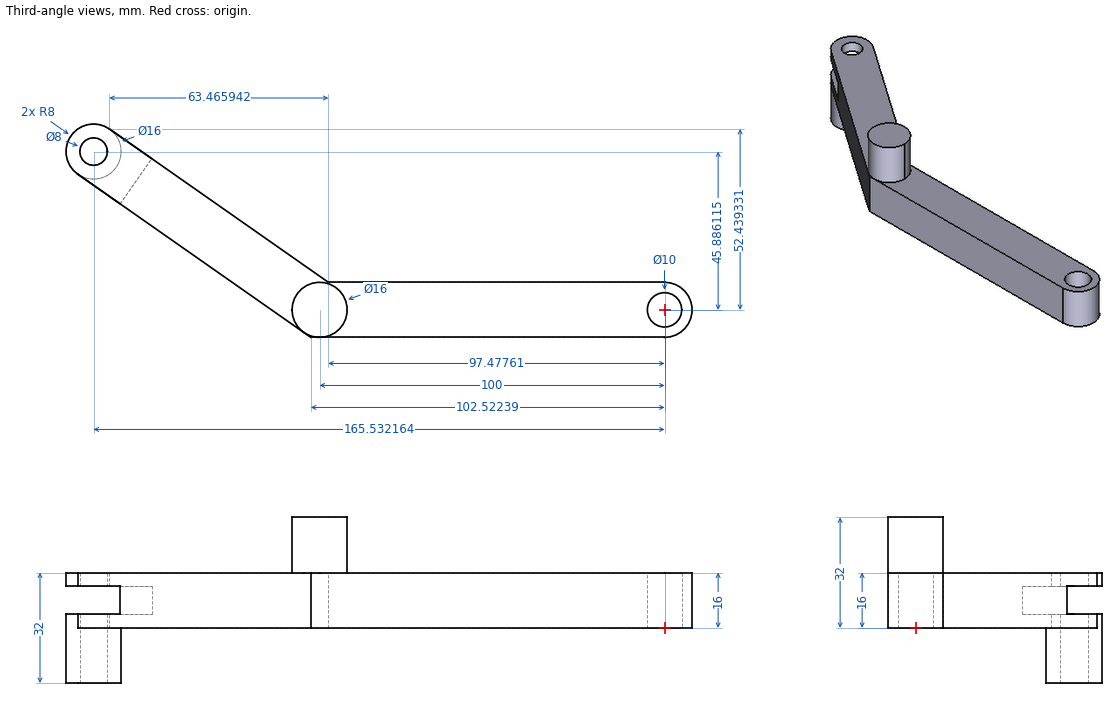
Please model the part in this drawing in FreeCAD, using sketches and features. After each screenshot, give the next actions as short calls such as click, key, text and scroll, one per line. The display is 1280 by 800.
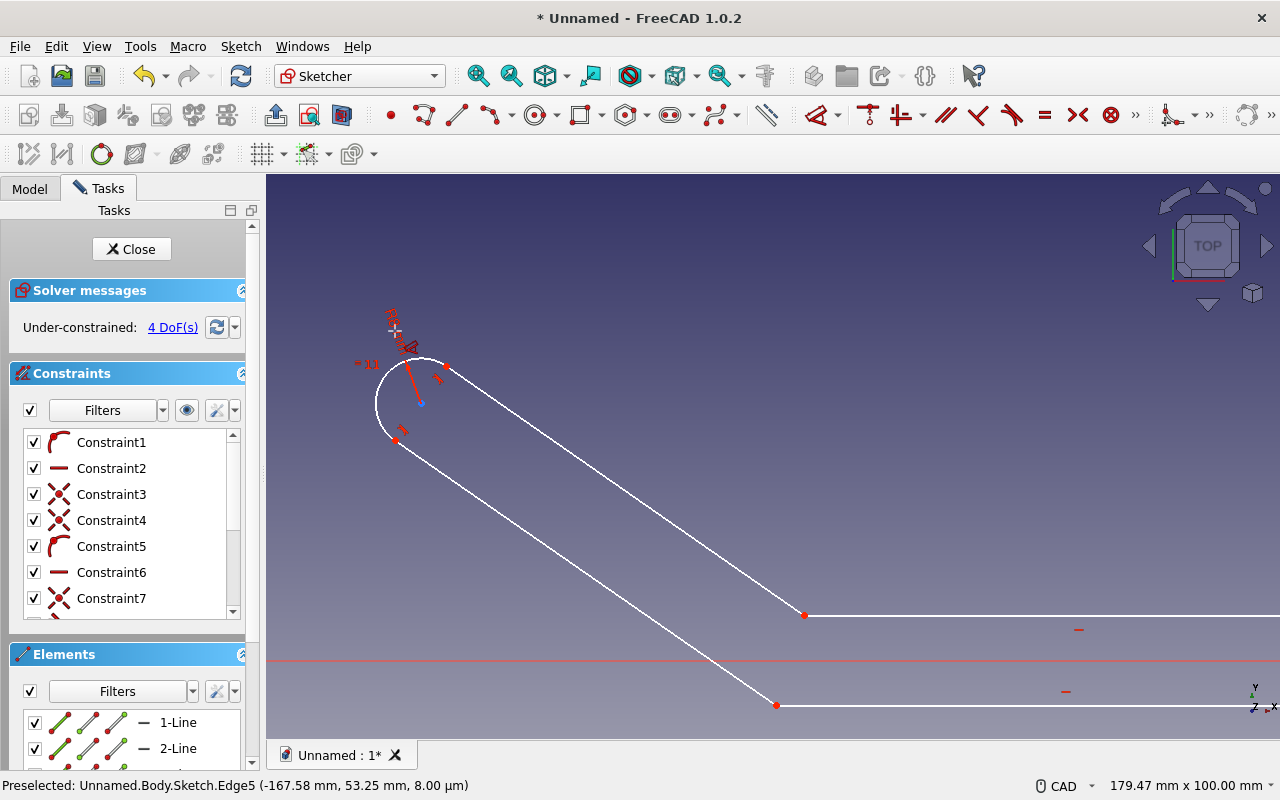
click(970, 616)
click(960, 582)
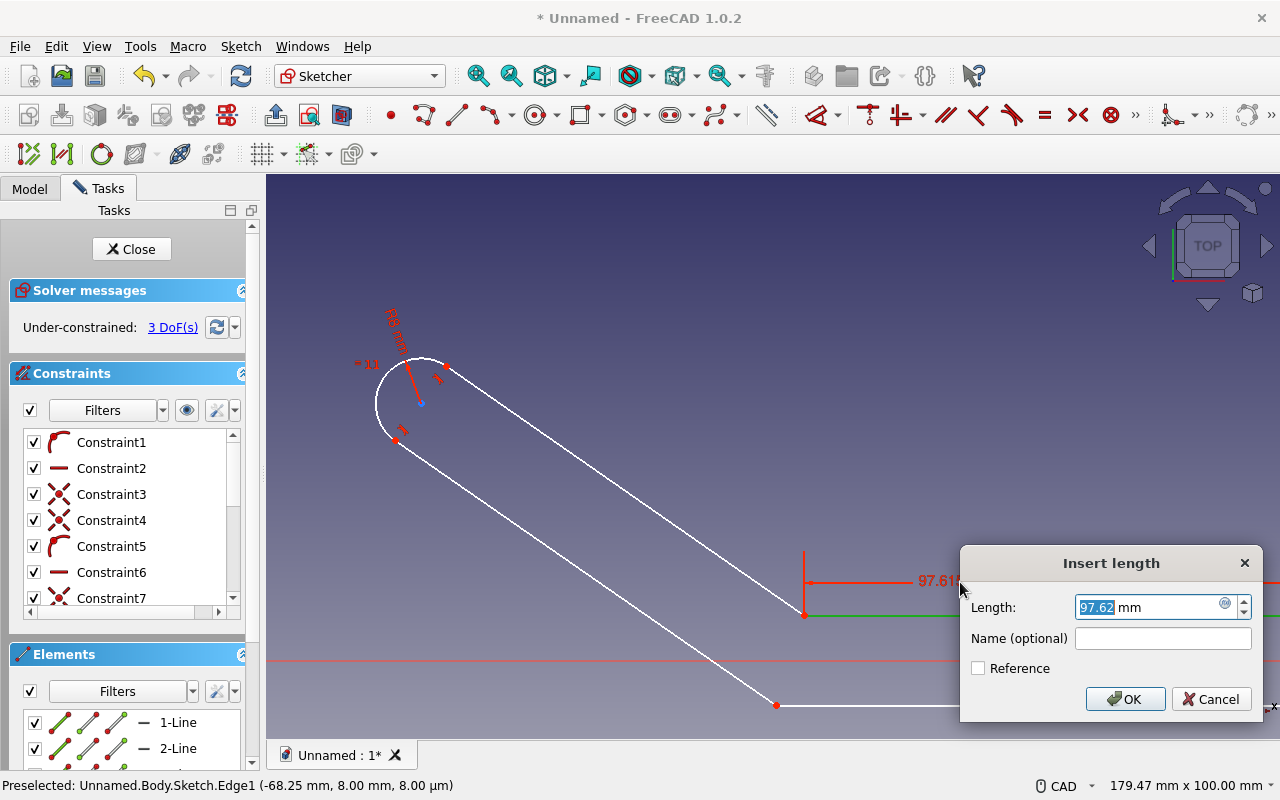
text(97.47761)
key(Return)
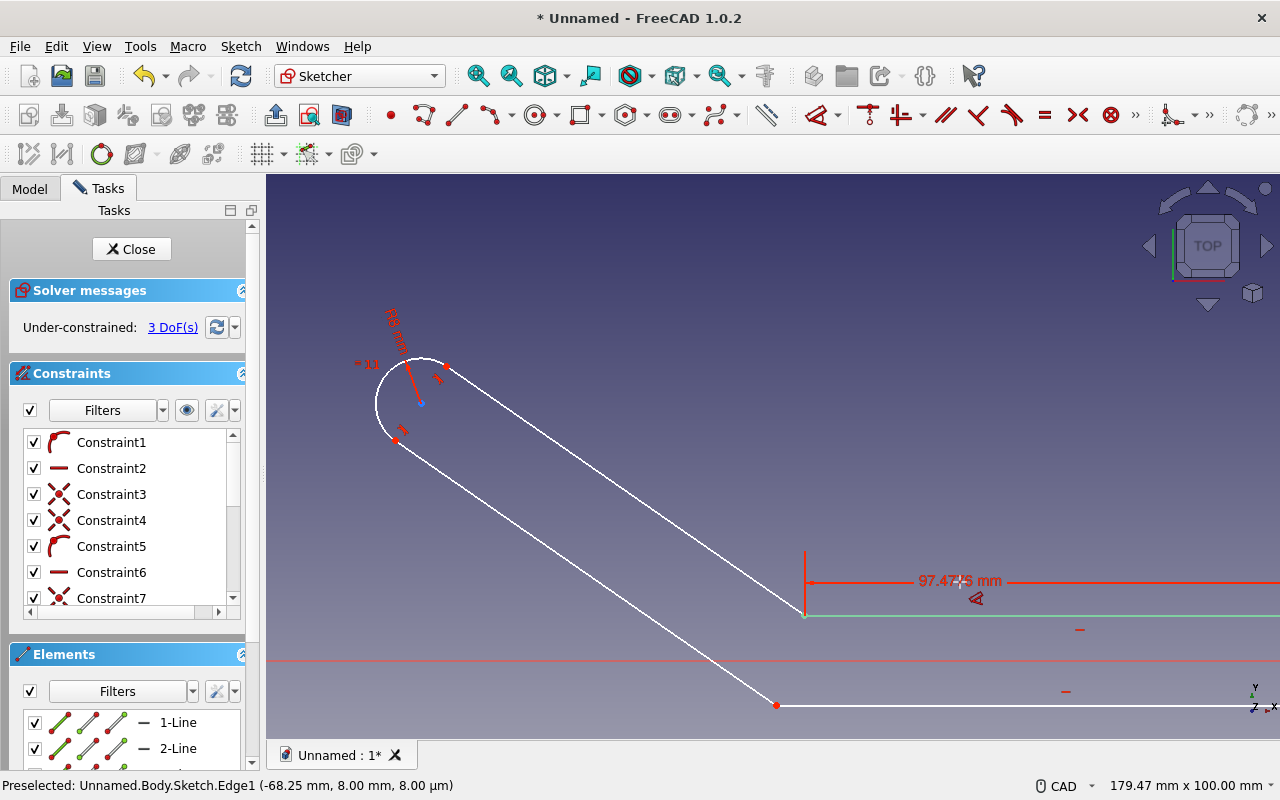
click(950, 706)
click(868, 600)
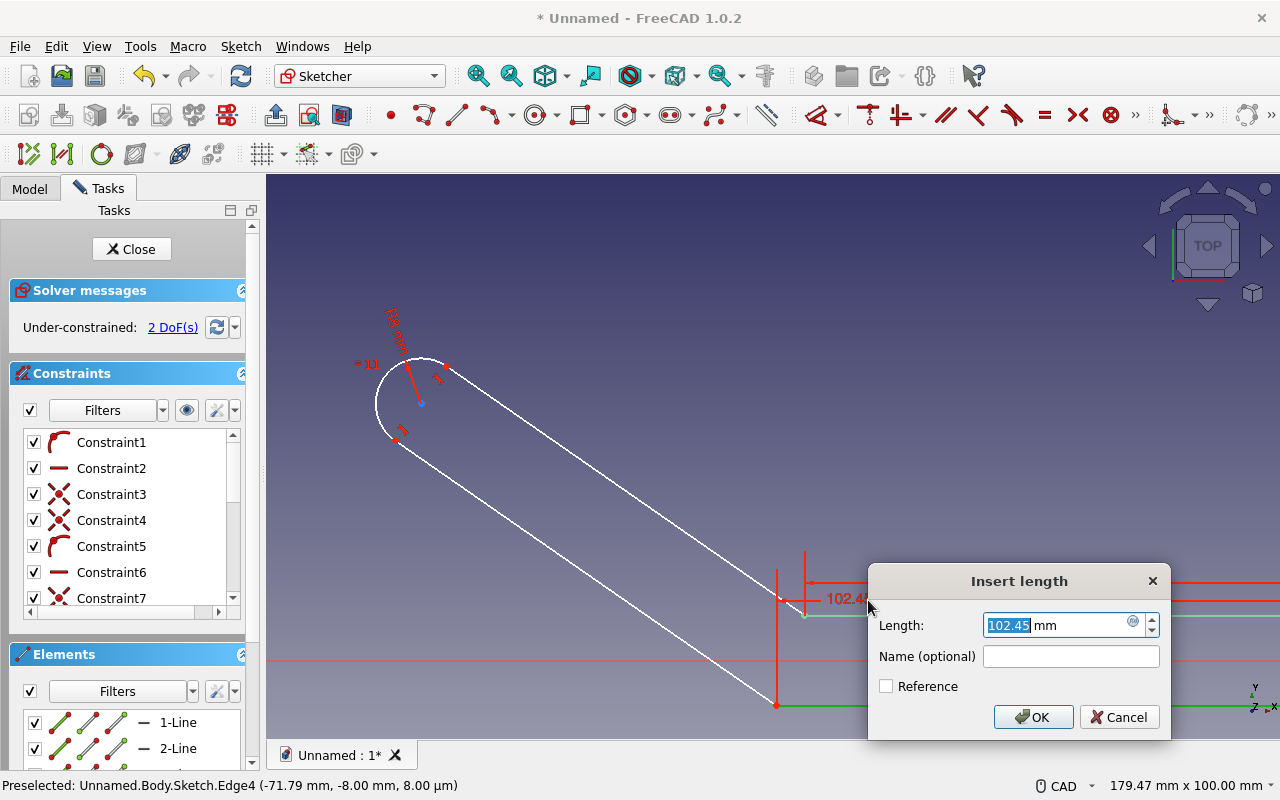
text(102.52239)
key(Return)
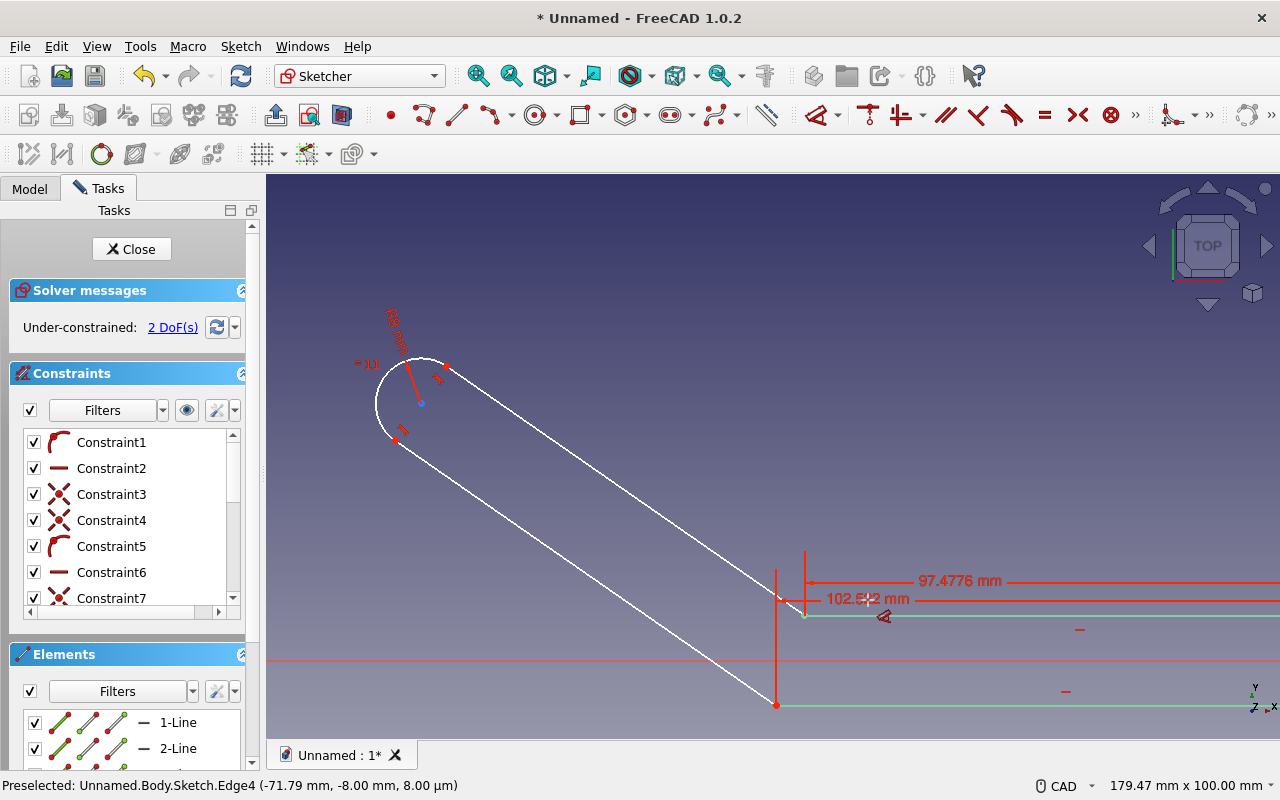
click(447, 367)
click(413, 514)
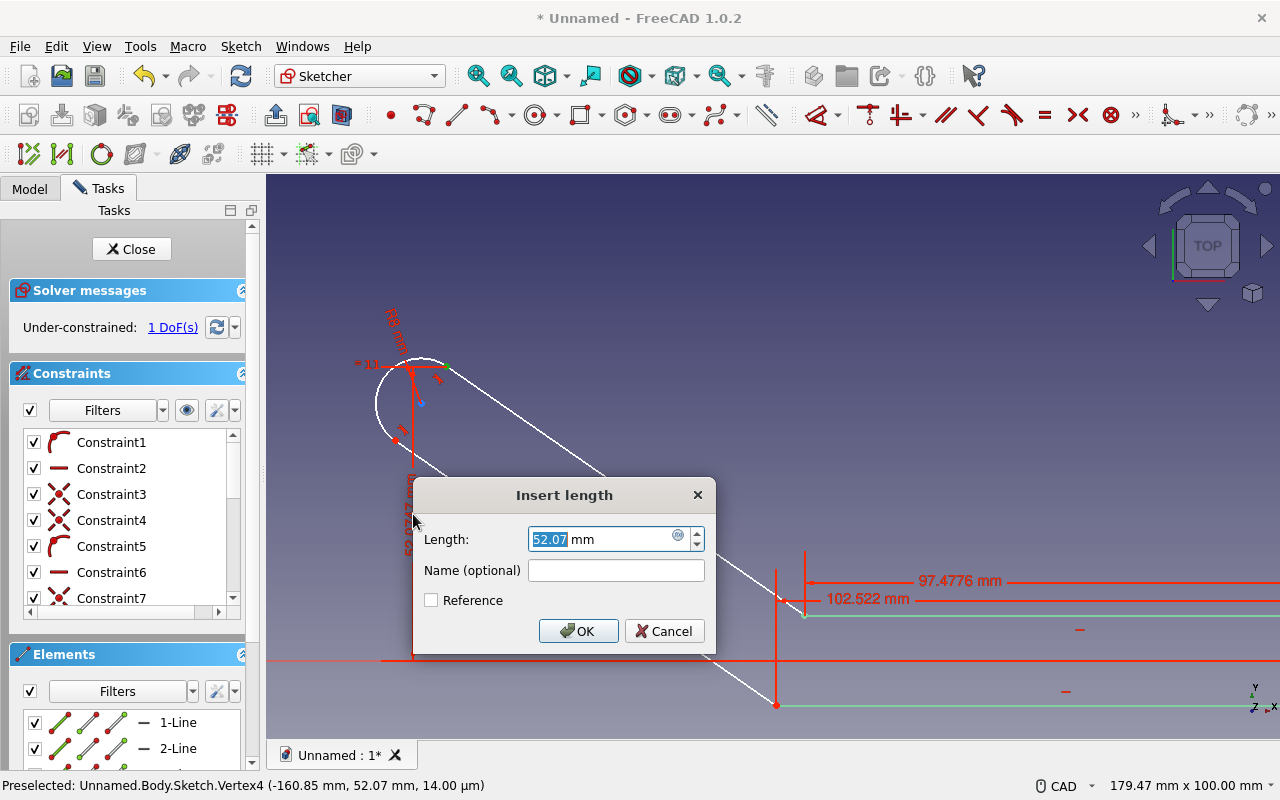
text(52.439331)
key(Return)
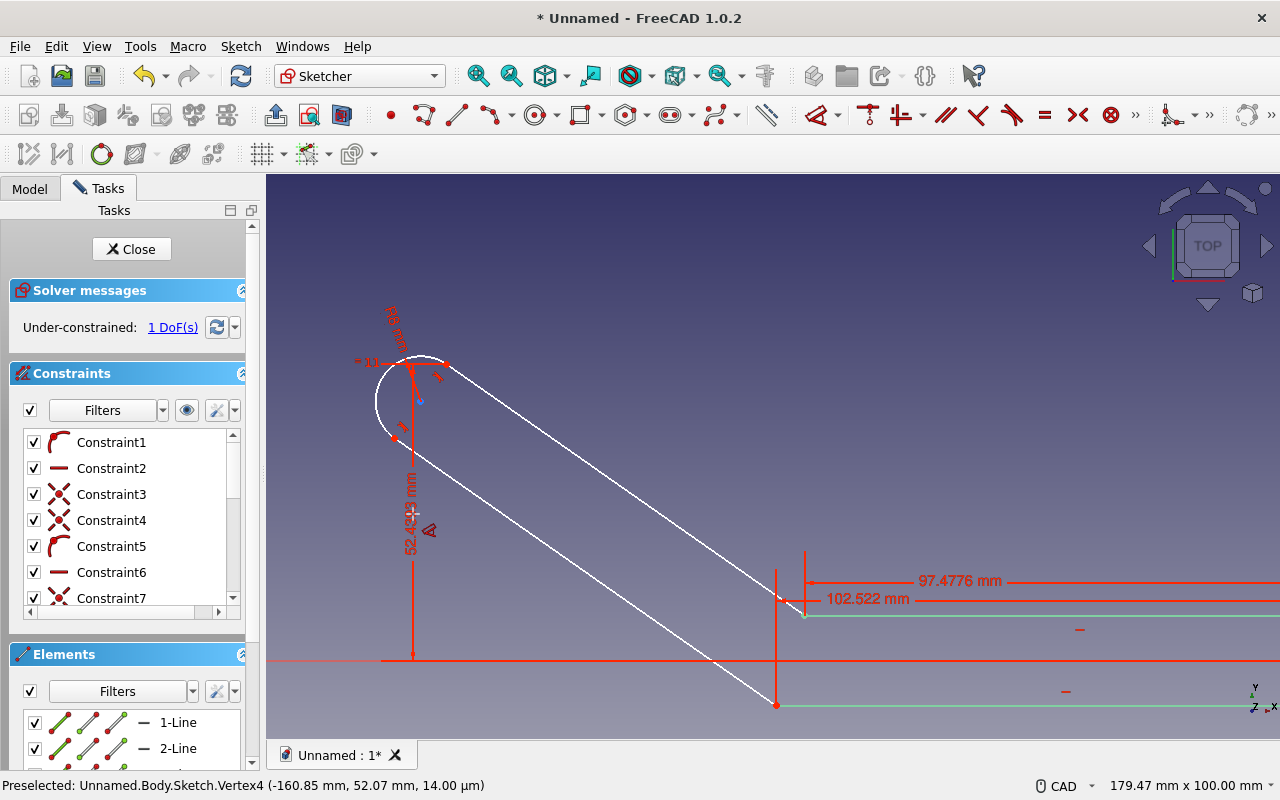
click(697, 540)
click(626, 330)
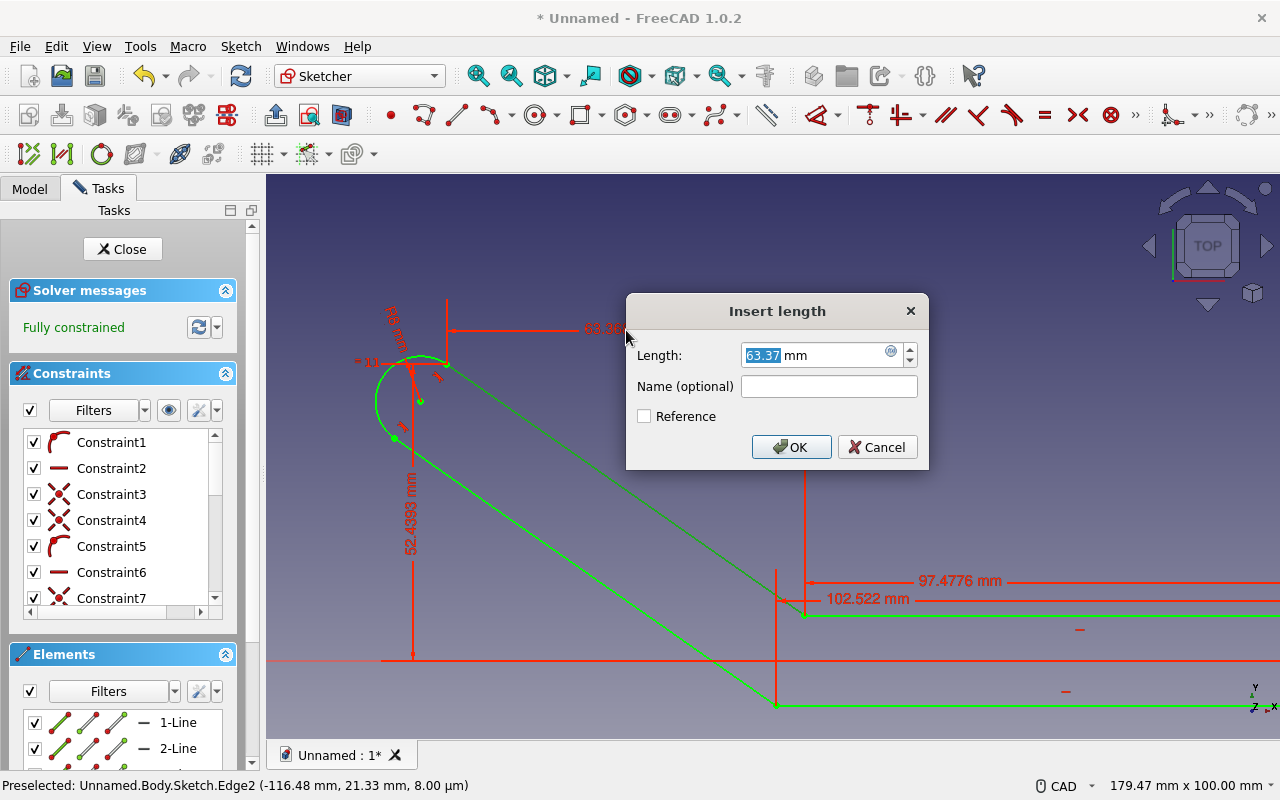
text(63.465942)
key(Return)
key(Escape)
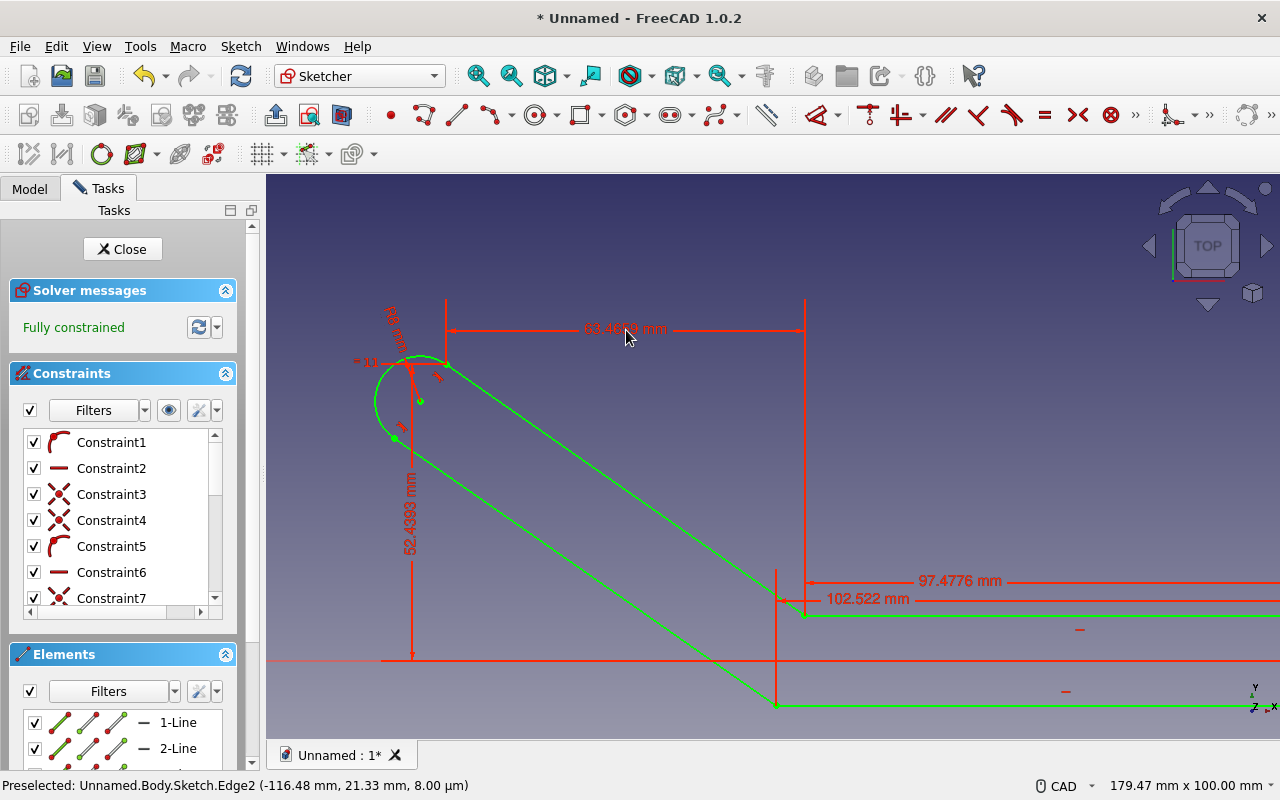
click(123, 249)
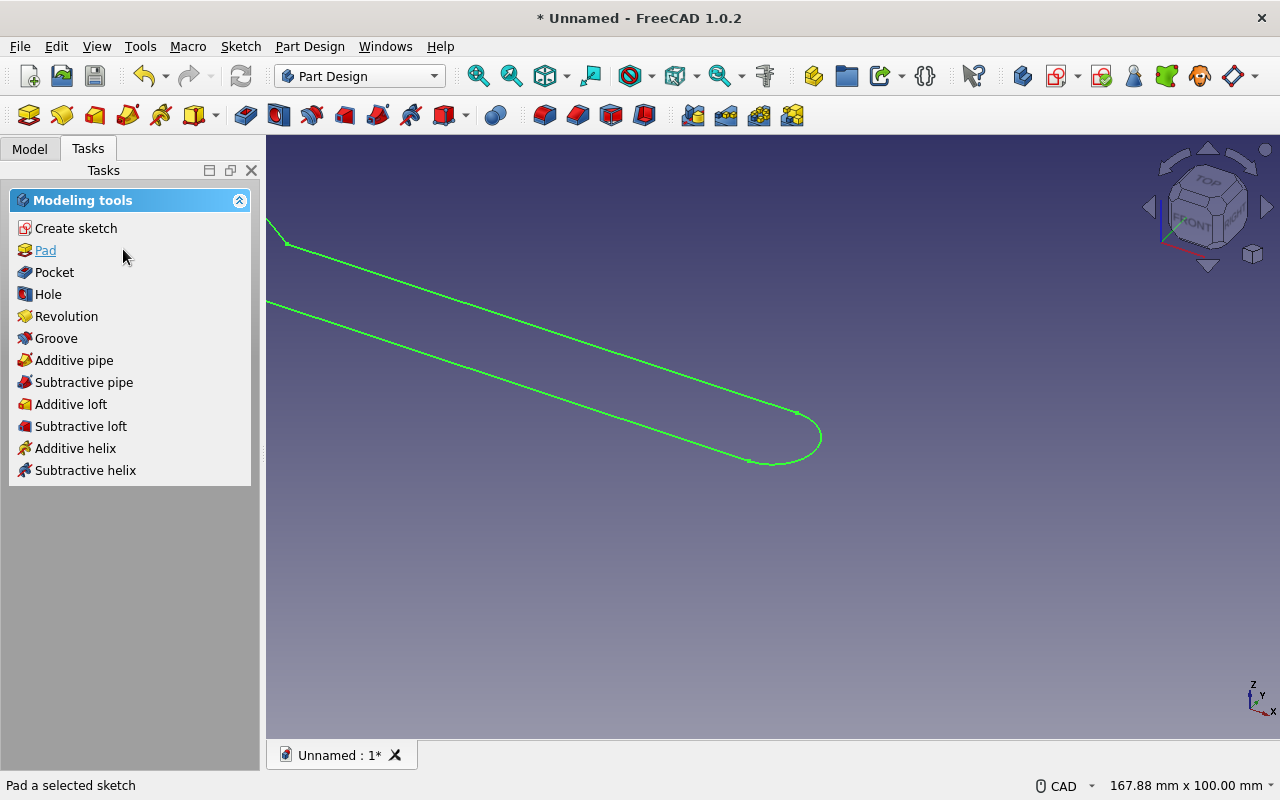
click(29, 116)